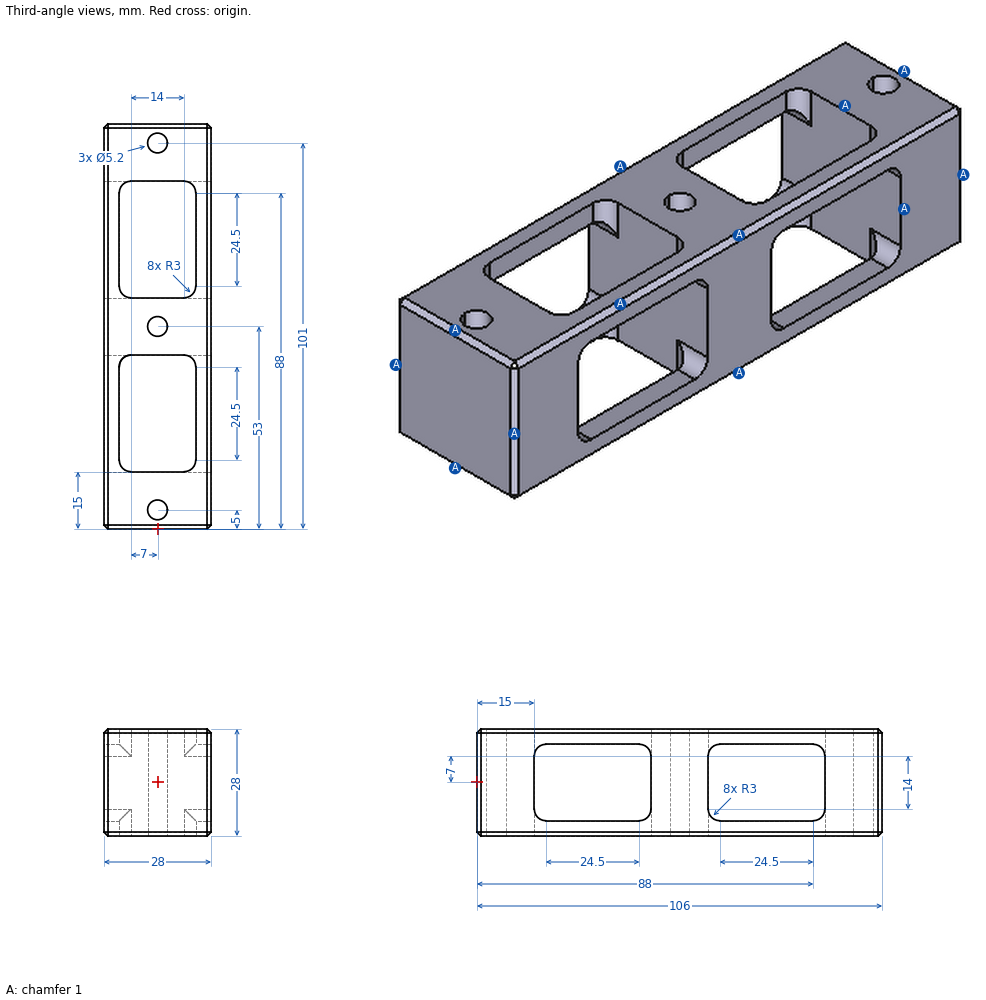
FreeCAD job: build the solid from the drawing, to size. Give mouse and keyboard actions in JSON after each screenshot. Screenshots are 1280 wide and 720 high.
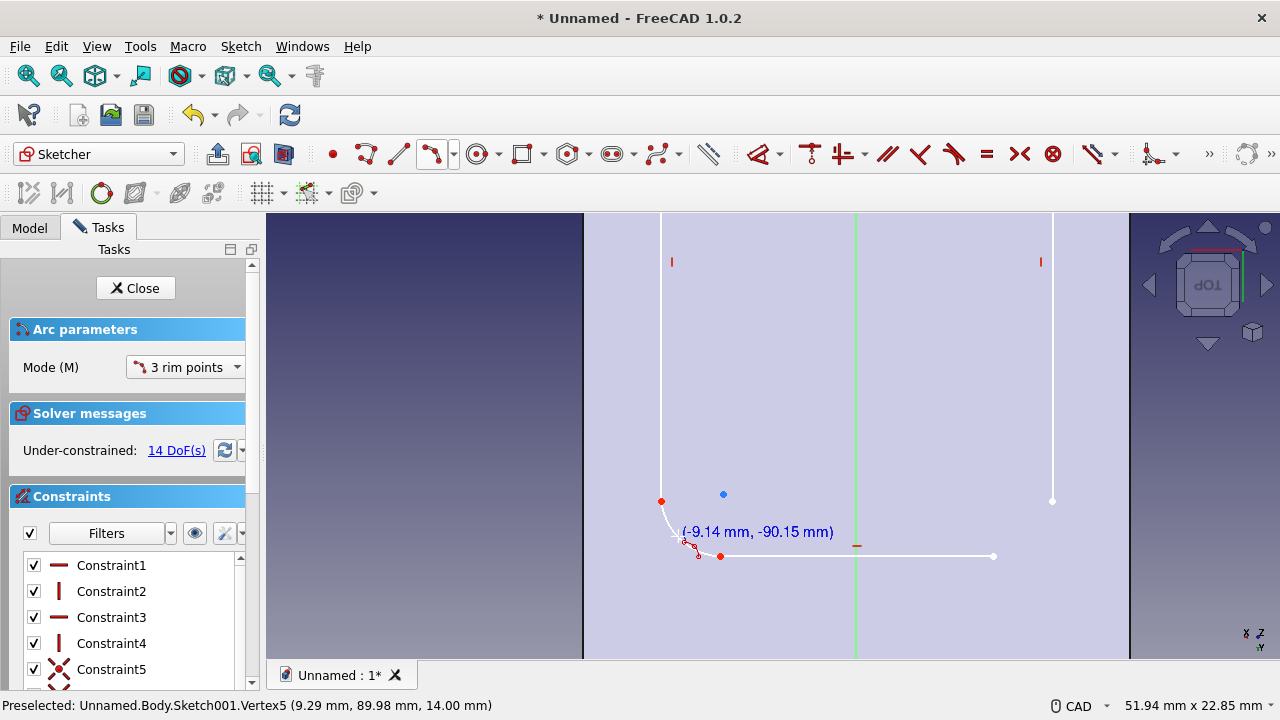
{"action": "scroll", "coordinate": [681, 537], "scroll_direction": "down", "scroll_amount": 10}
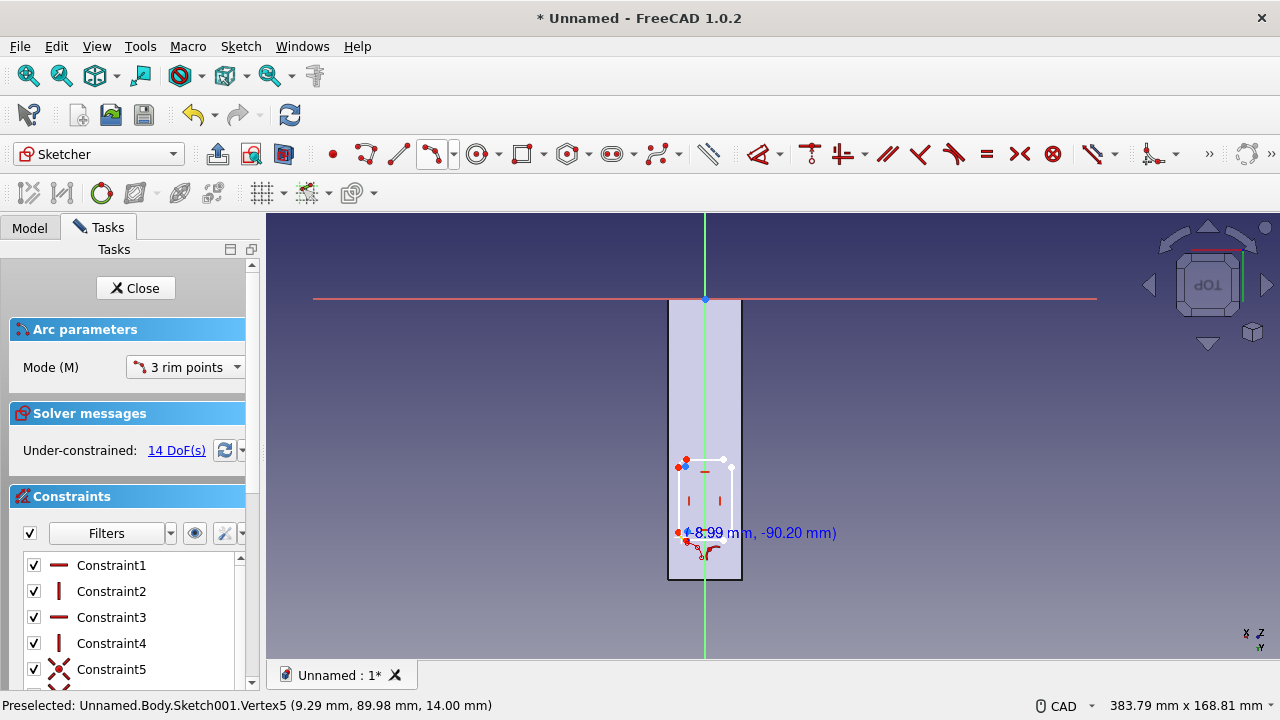
{"action": "scroll", "coordinate": [724, 540], "scroll_direction": "up", "scroll_amount": 2}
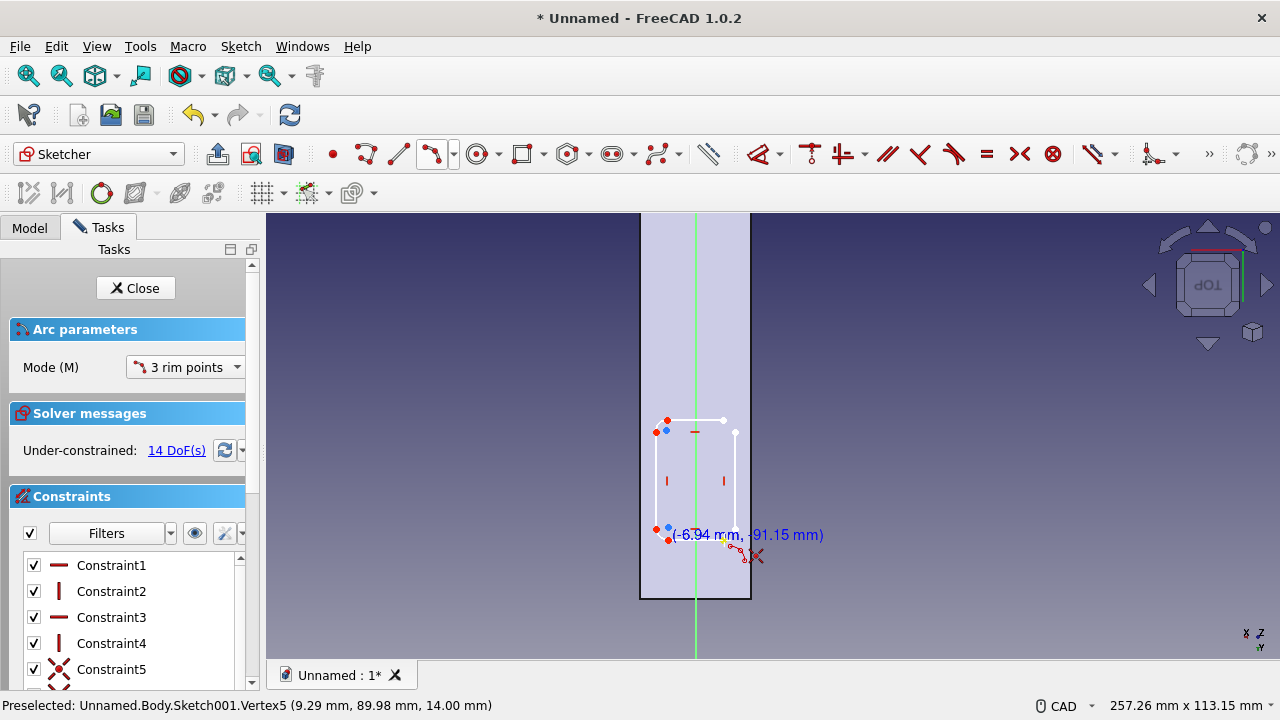
{"action": "left_click", "coordinate": [723, 540]}
{"action": "left_click", "coordinate": [735, 529]}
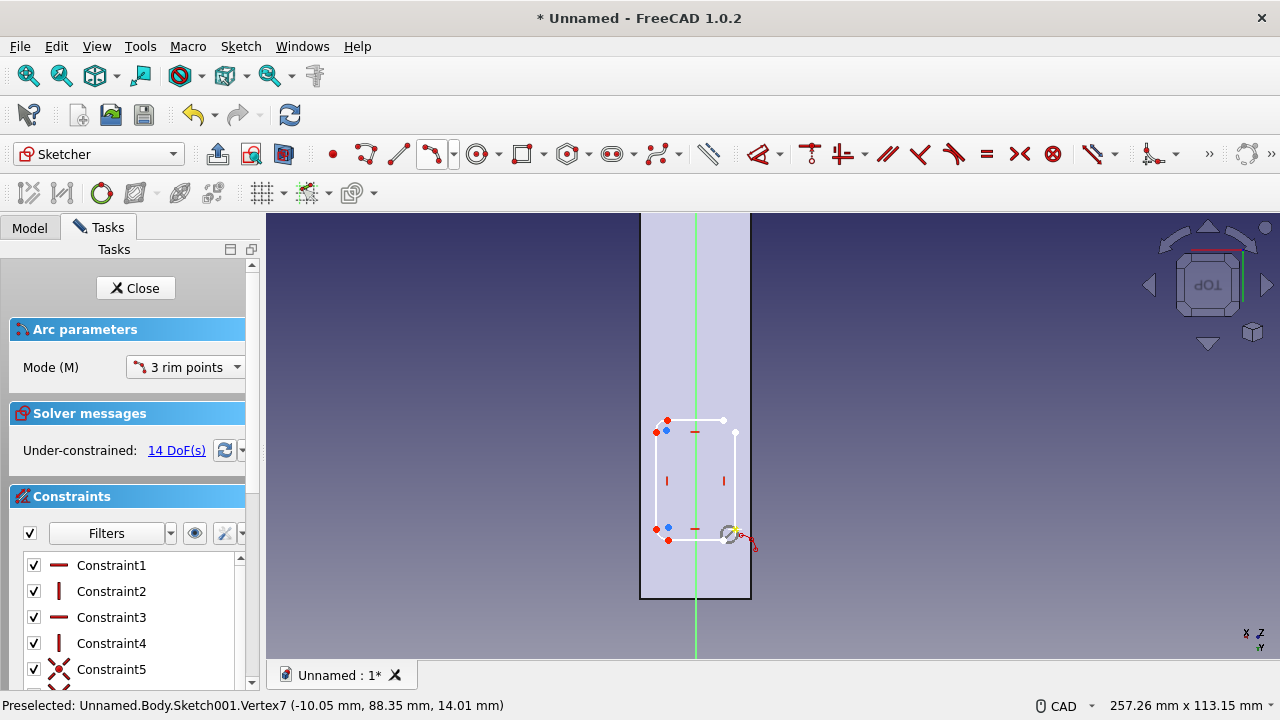
{"action": "scroll", "coordinate": [732, 536], "scroll_direction": "up", "scroll_amount": 8}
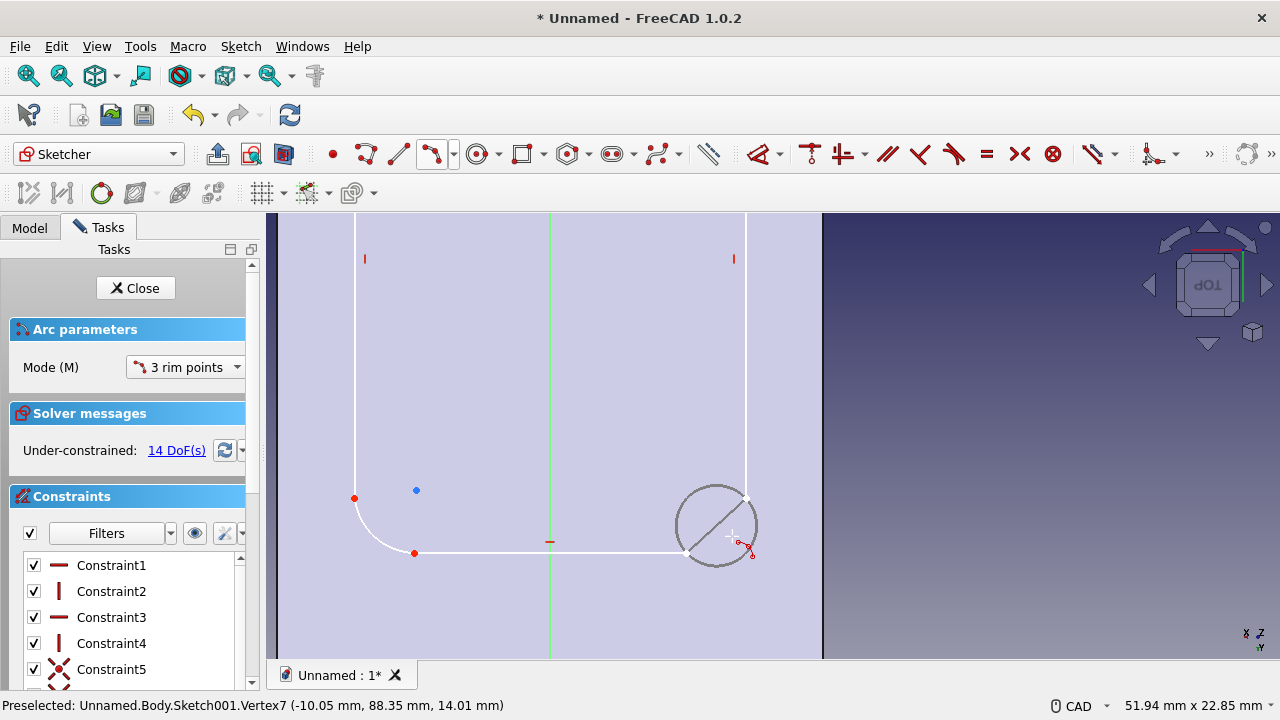
{"action": "left_click", "coordinate": [728, 533]}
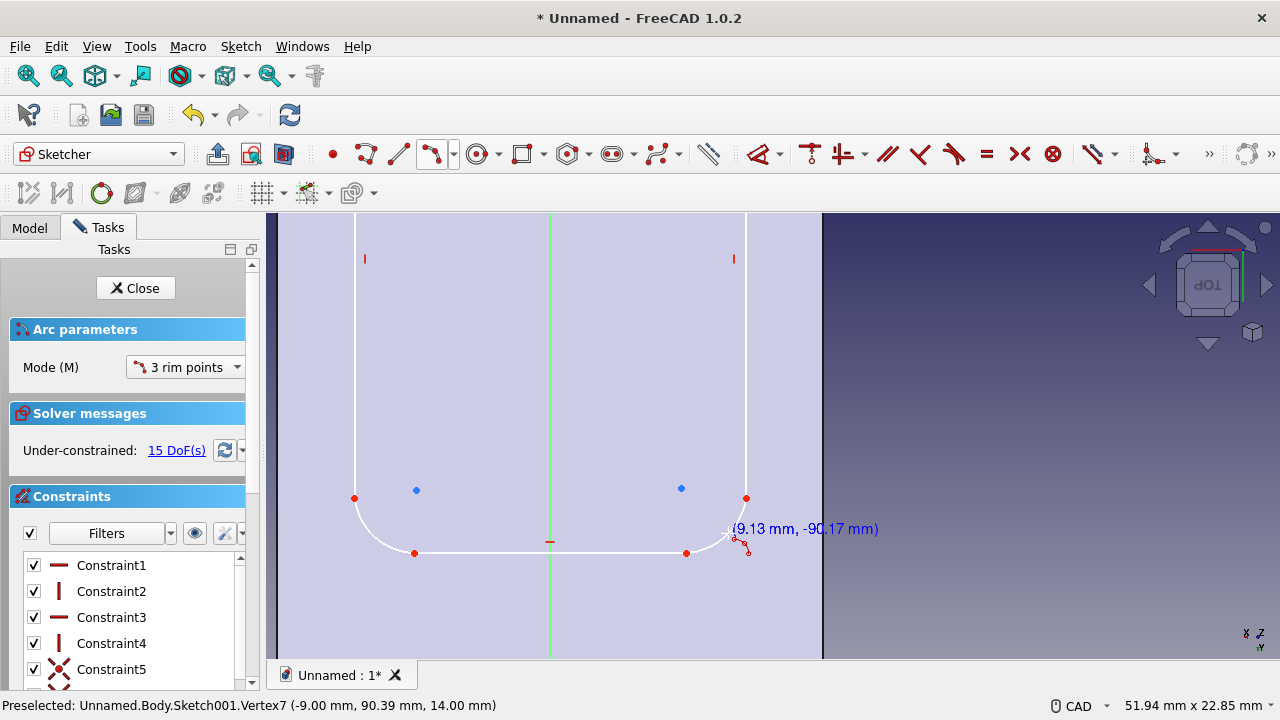
{"action": "scroll", "coordinate": [729, 538], "scroll_direction": "down", "scroll_amount": 10}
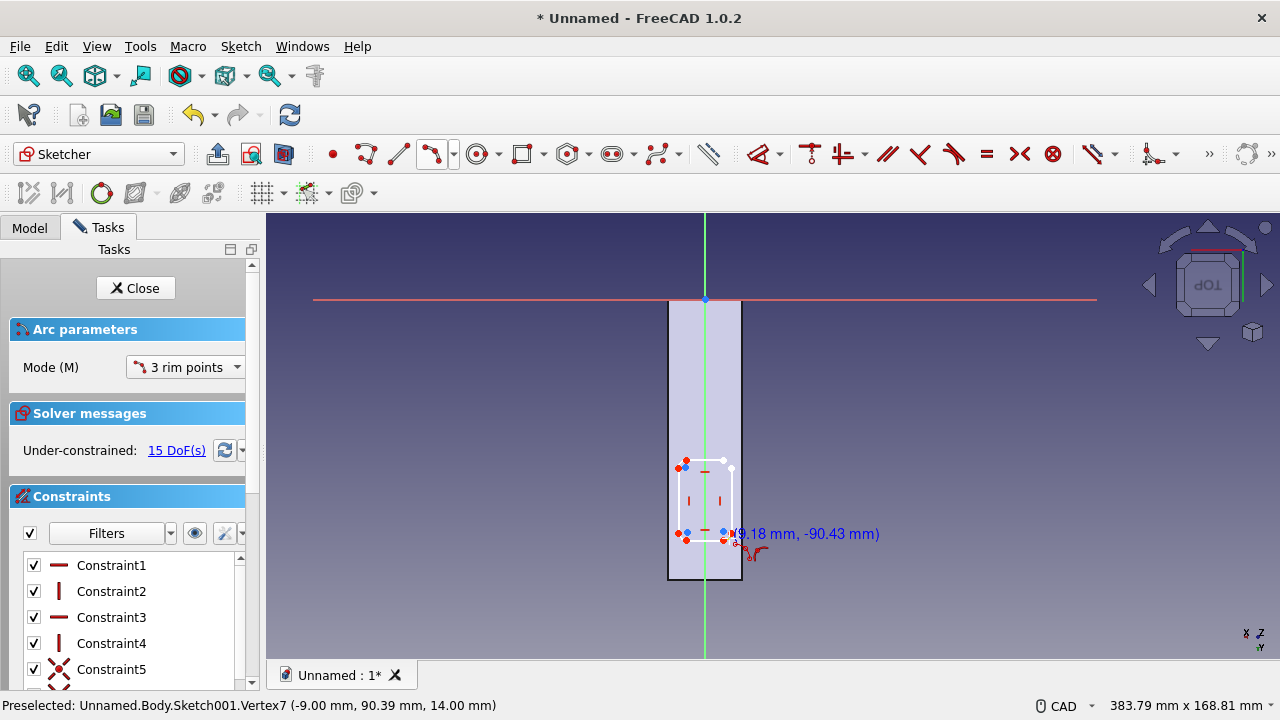
{"action": "scroll", "coordinate": [732, 468], "scroll_direction": "up", "scroll_amount": 2}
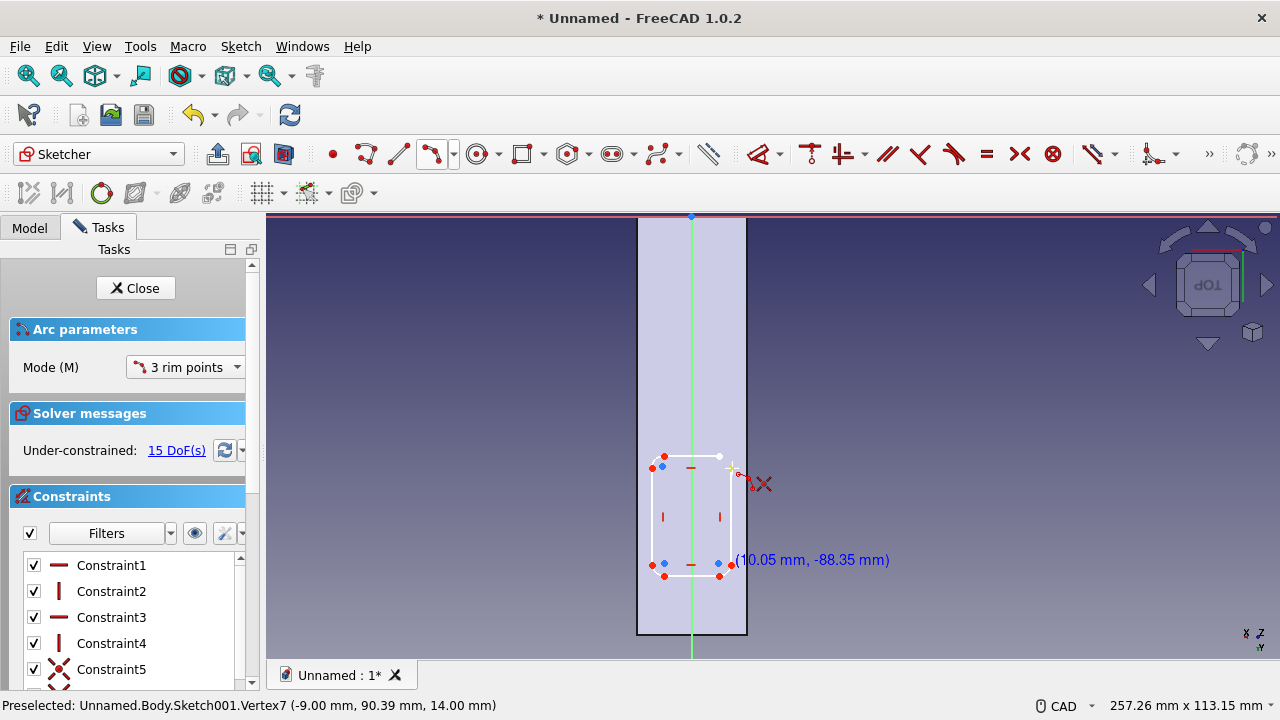
{"action": "left_click", "coordinate": [731, 468]}
{"action": "left_click", "coordinate": [719, 456]}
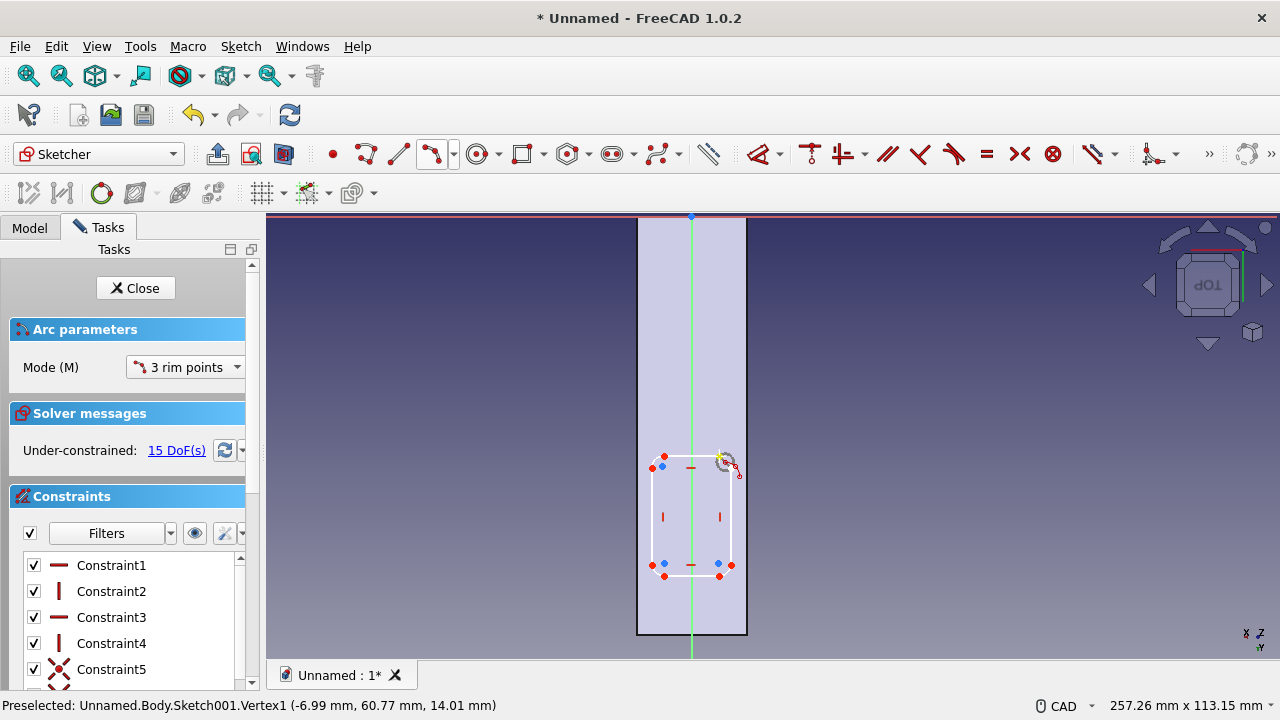
{"action": "scroll", "coordinate": [728, 459], "scroll_direction": "up", "scroll_amount": 8}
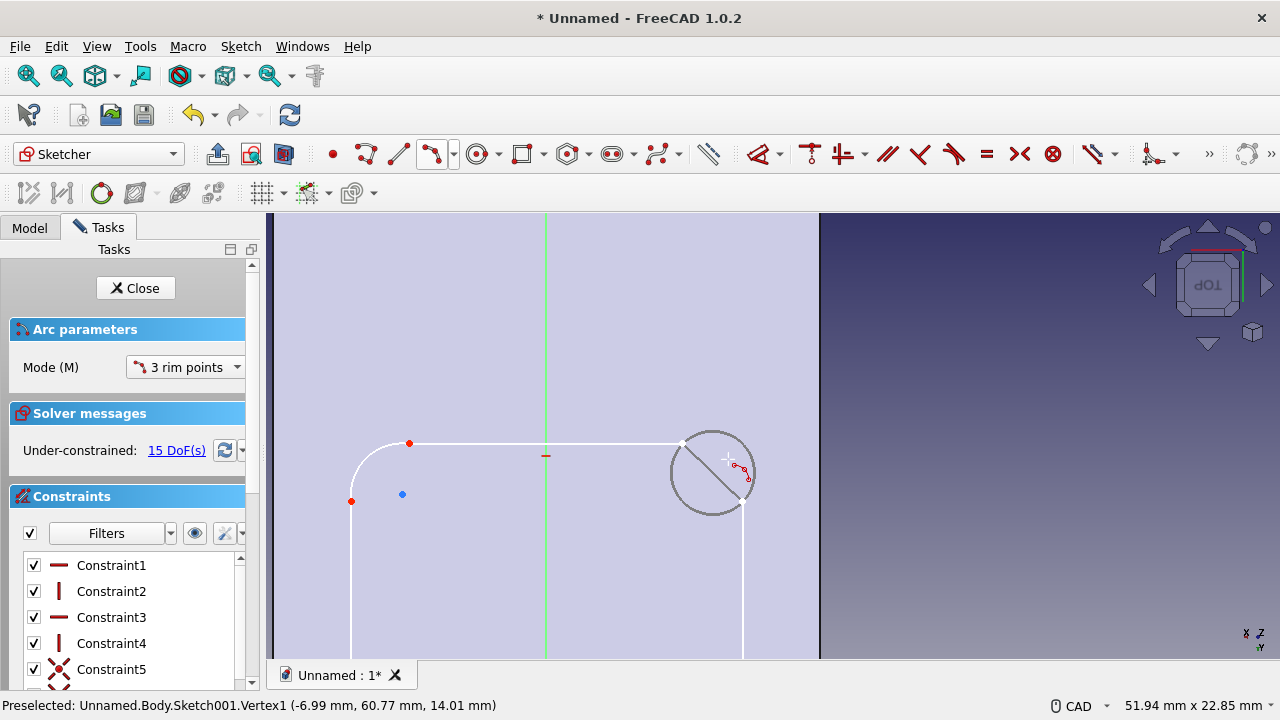
{"action": "left_click", "coordinate": [725, 456]}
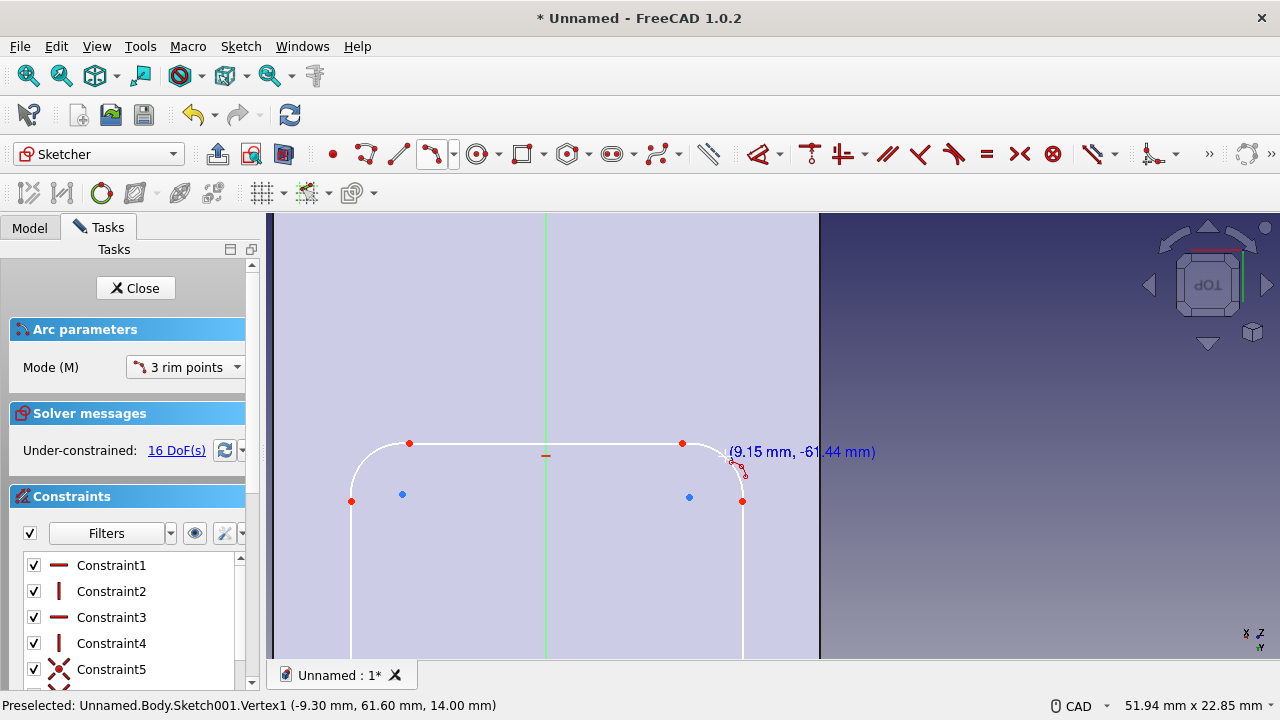
{"action": "key", "text": "g l"}